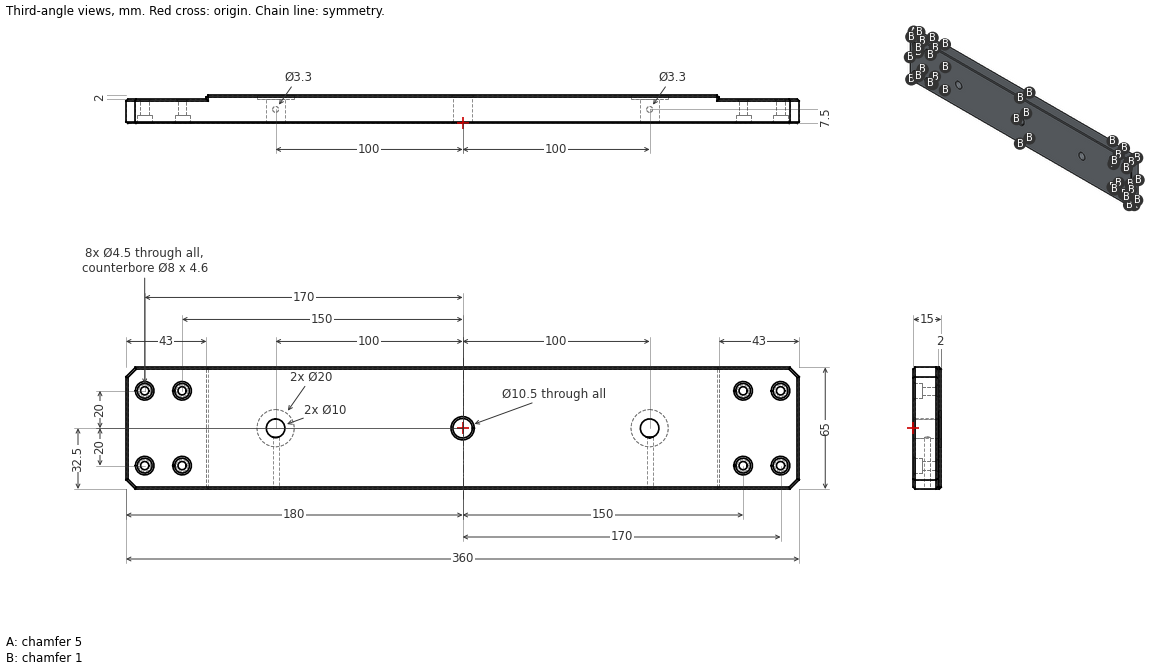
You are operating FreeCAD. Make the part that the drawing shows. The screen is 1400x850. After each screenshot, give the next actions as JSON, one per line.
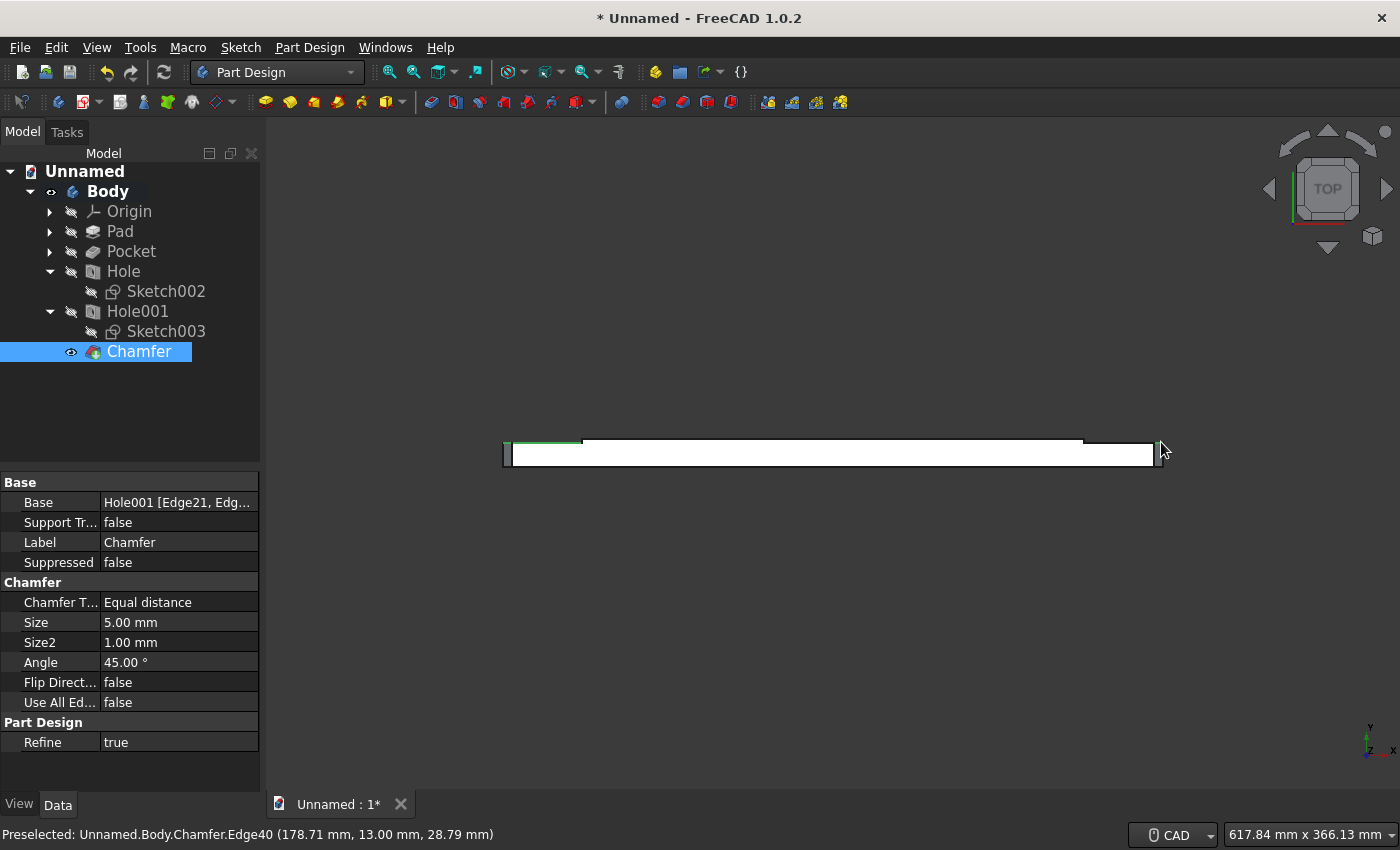
{"action": "left_click", "coordinate": [1119, 442], "text": "ctrl"}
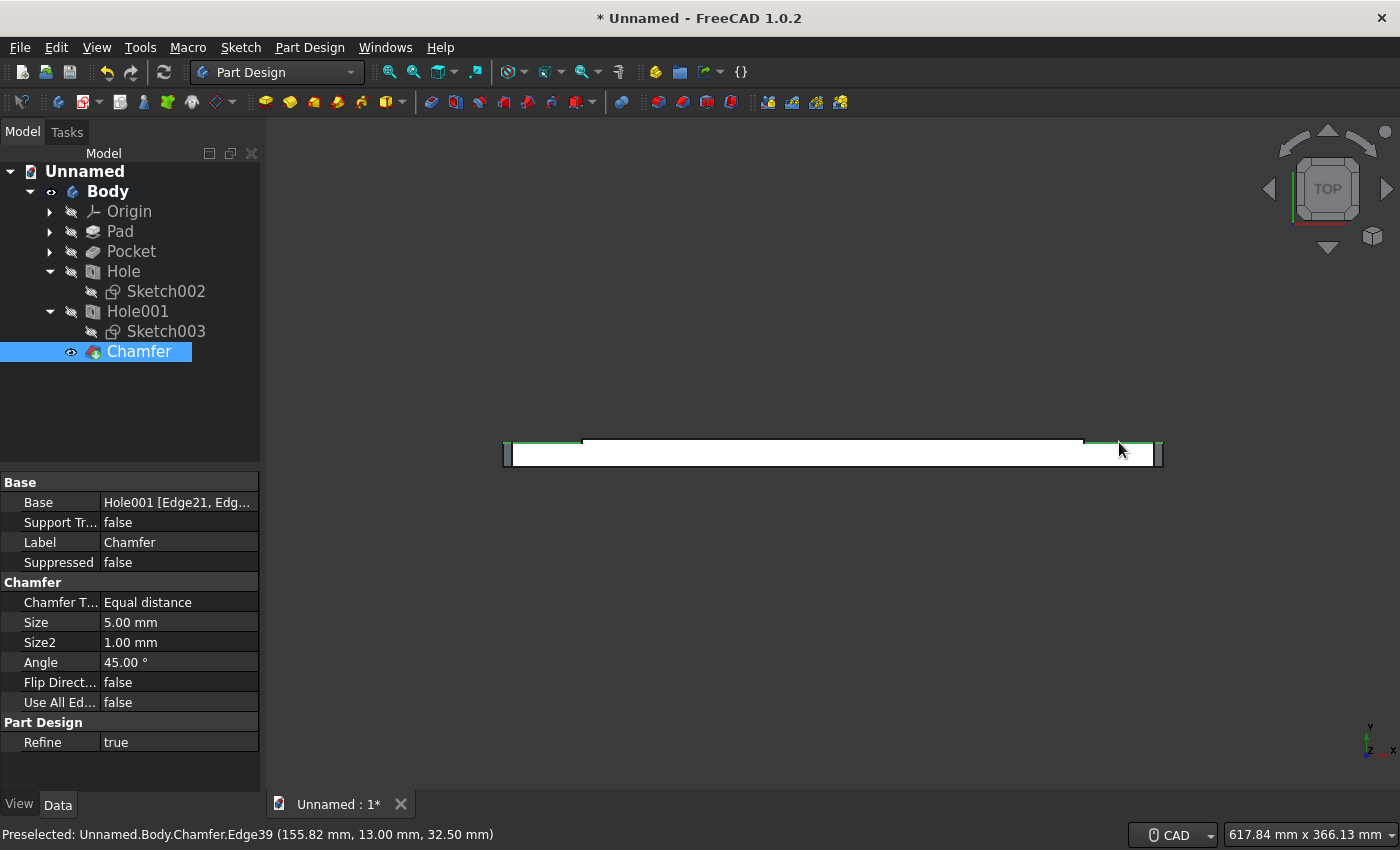
{"action": "key", "text": "1"}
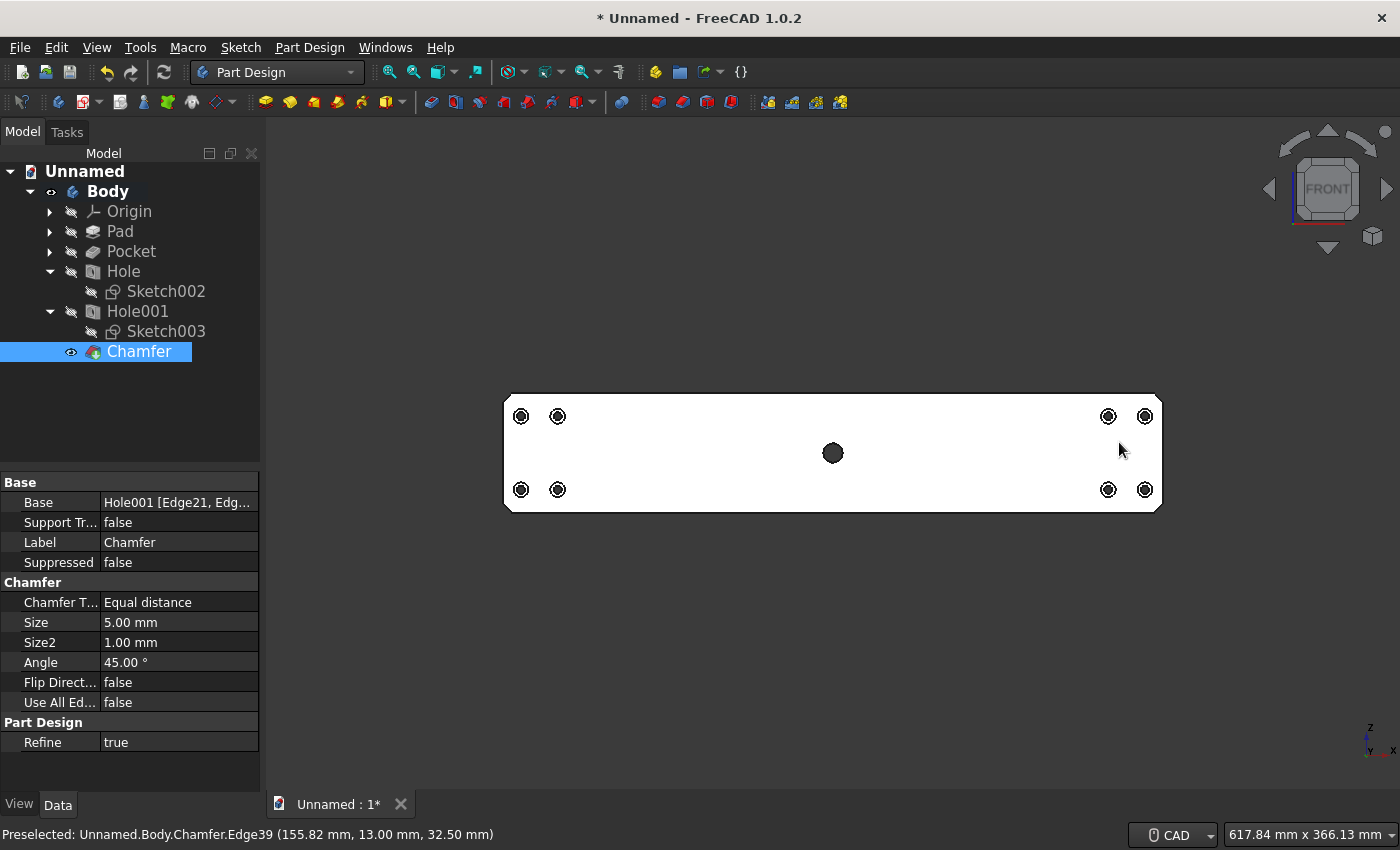
{"action": "key", "text": "3"}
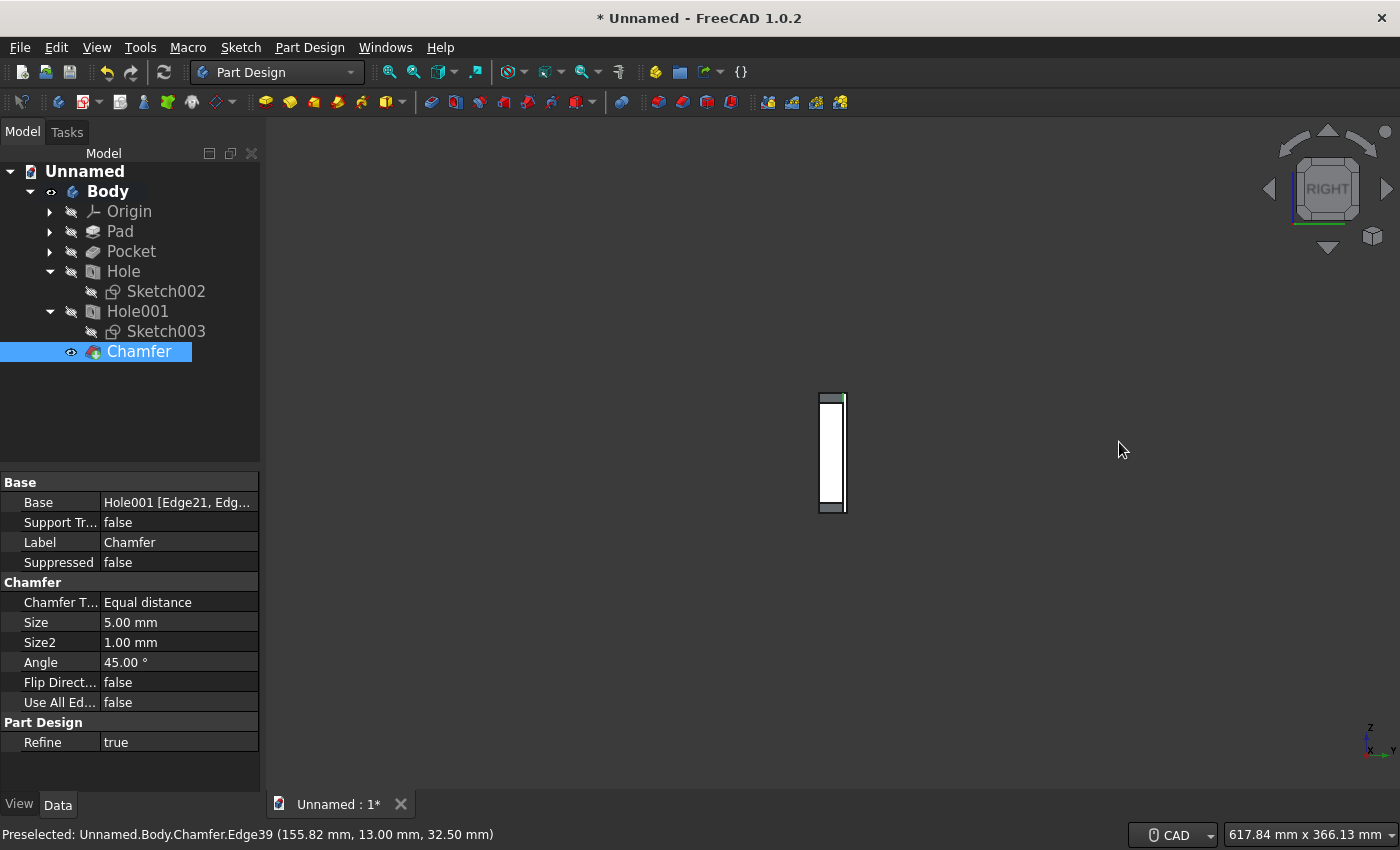
{"action": "left_click", "coordinate": [390, 72]}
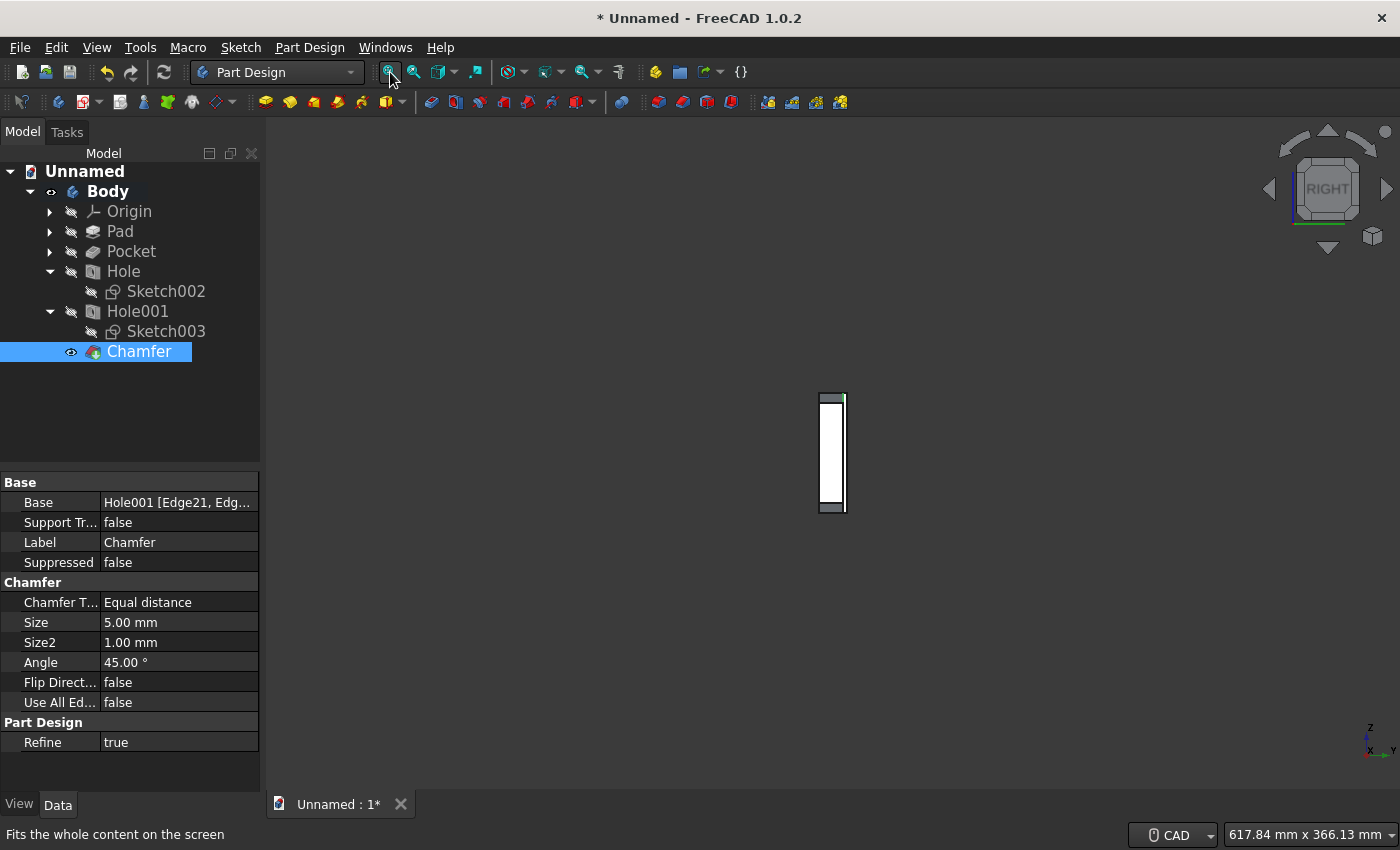
{"action": "left_click", "coordinate": [843, 452], "text": "ctrl"}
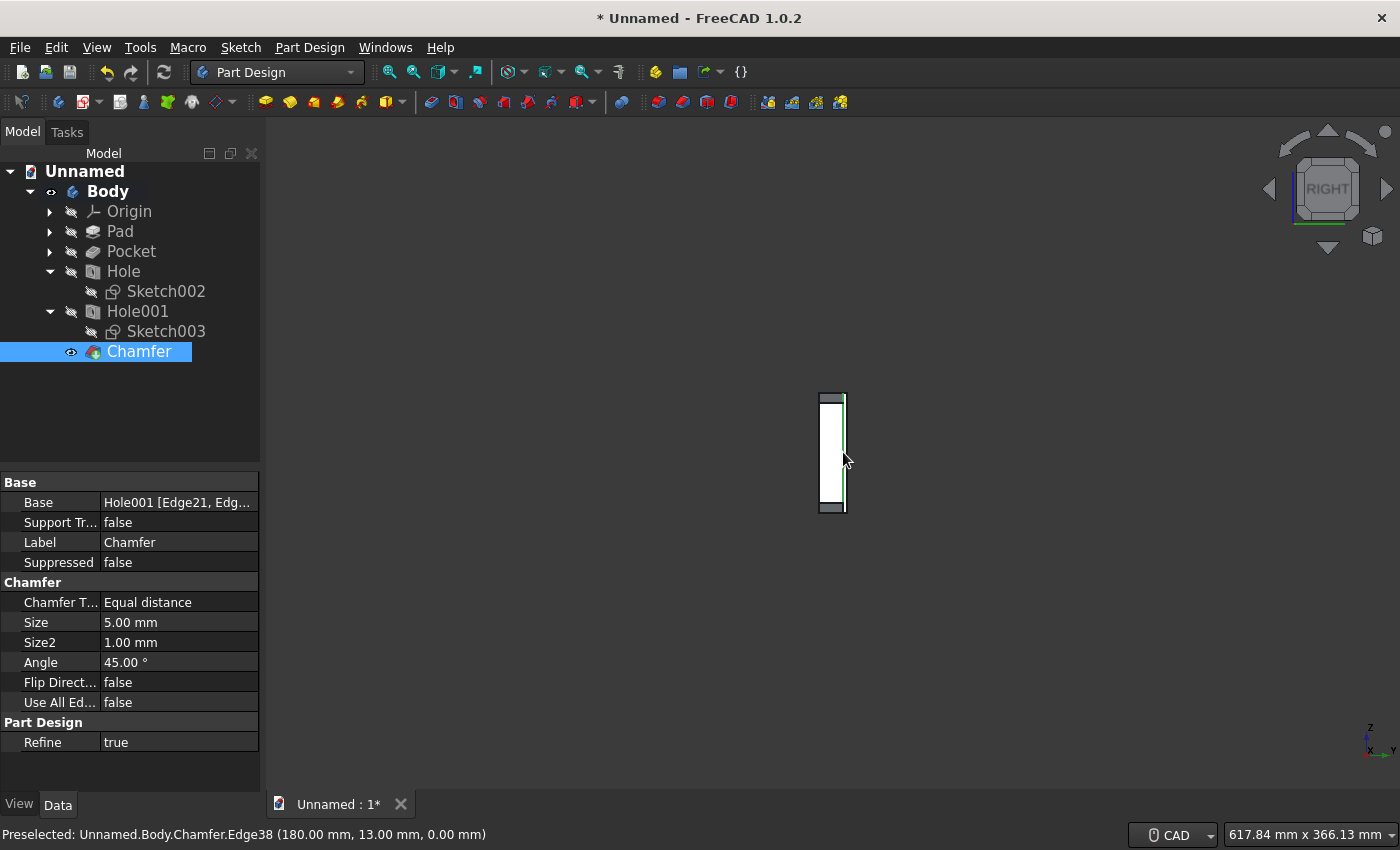
{"action": "left_click", "coordinate": [843, 509], "text": "ctrl"}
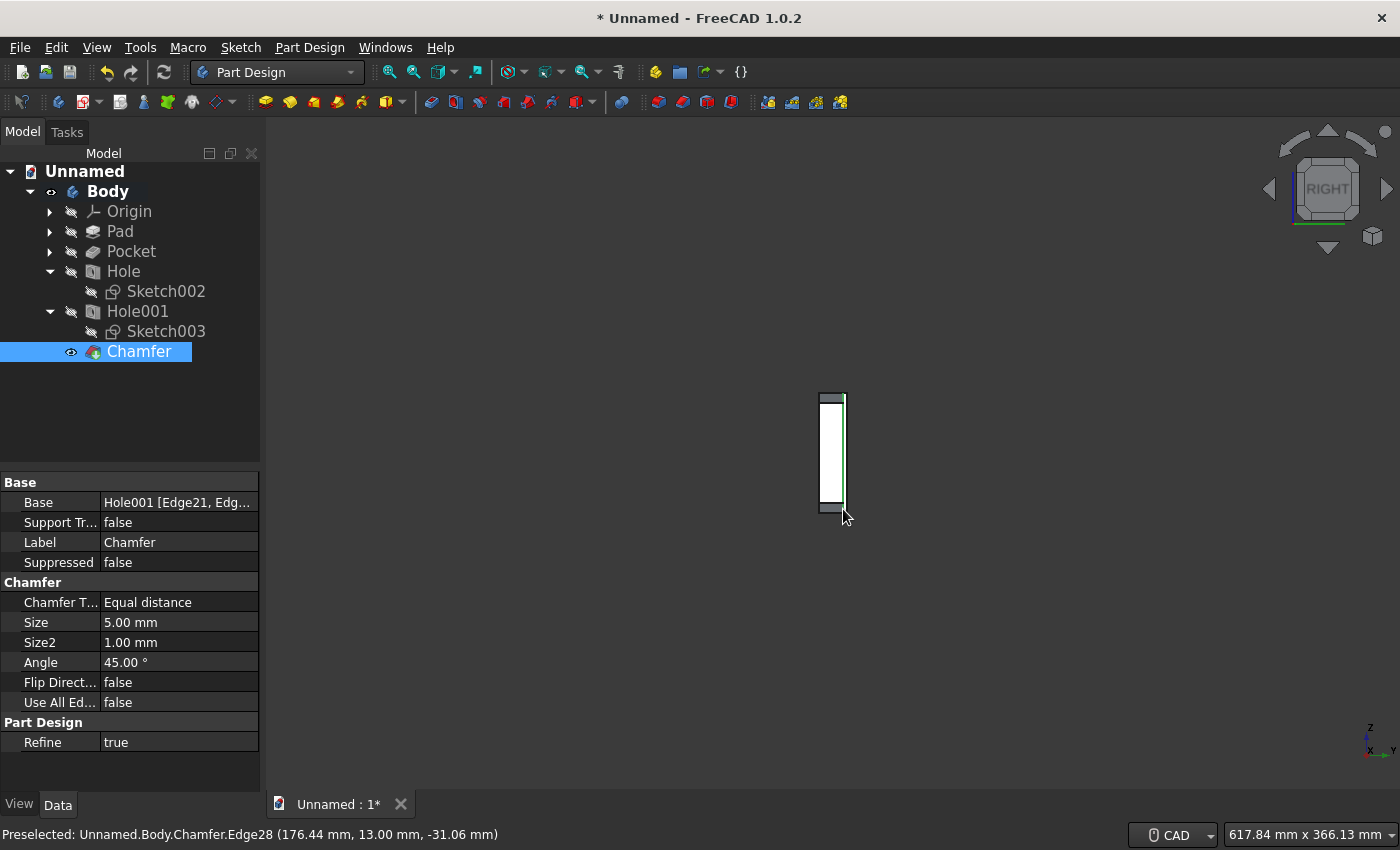
{"action": "key", "text": "5"}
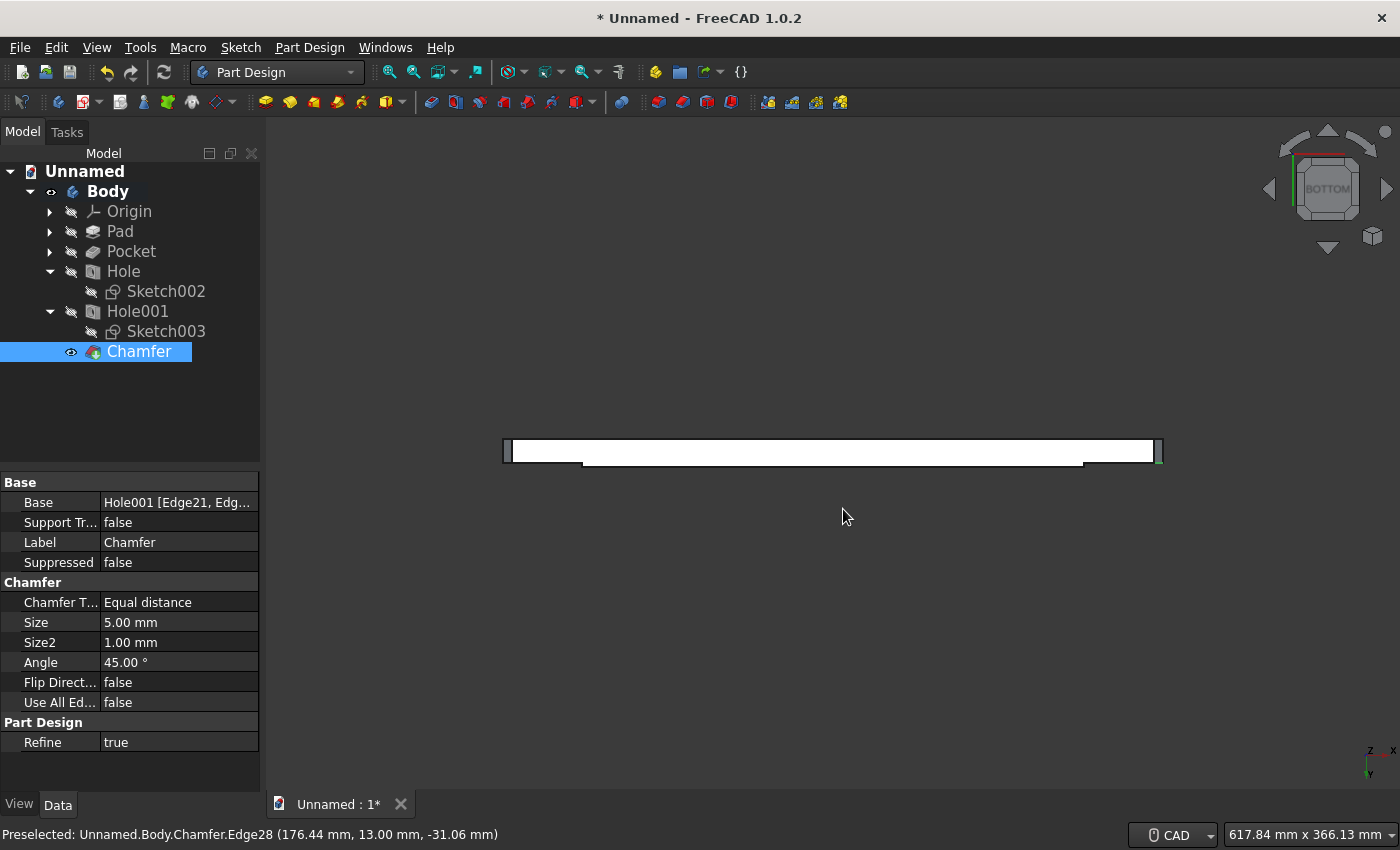
{"action": "key", "text": "4"}